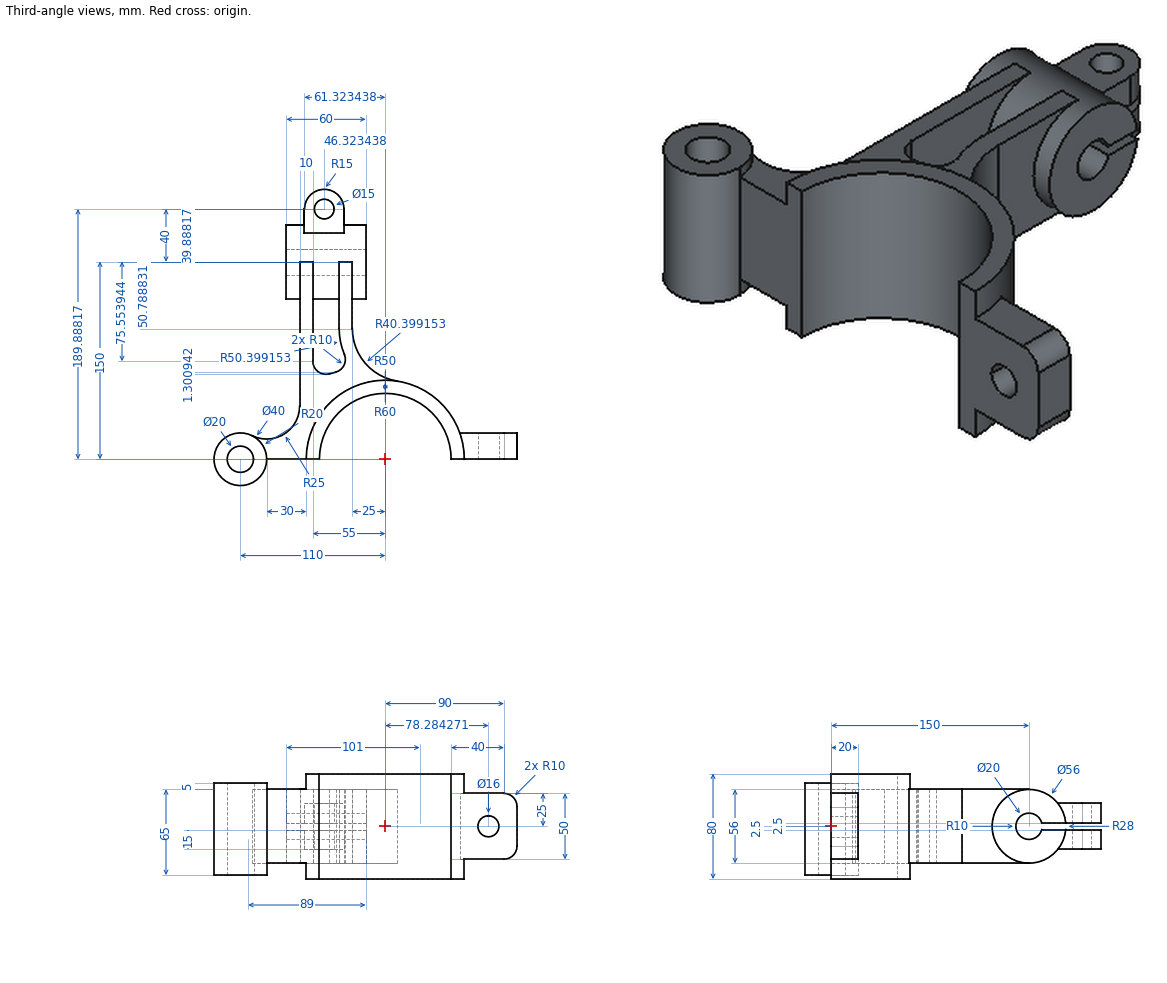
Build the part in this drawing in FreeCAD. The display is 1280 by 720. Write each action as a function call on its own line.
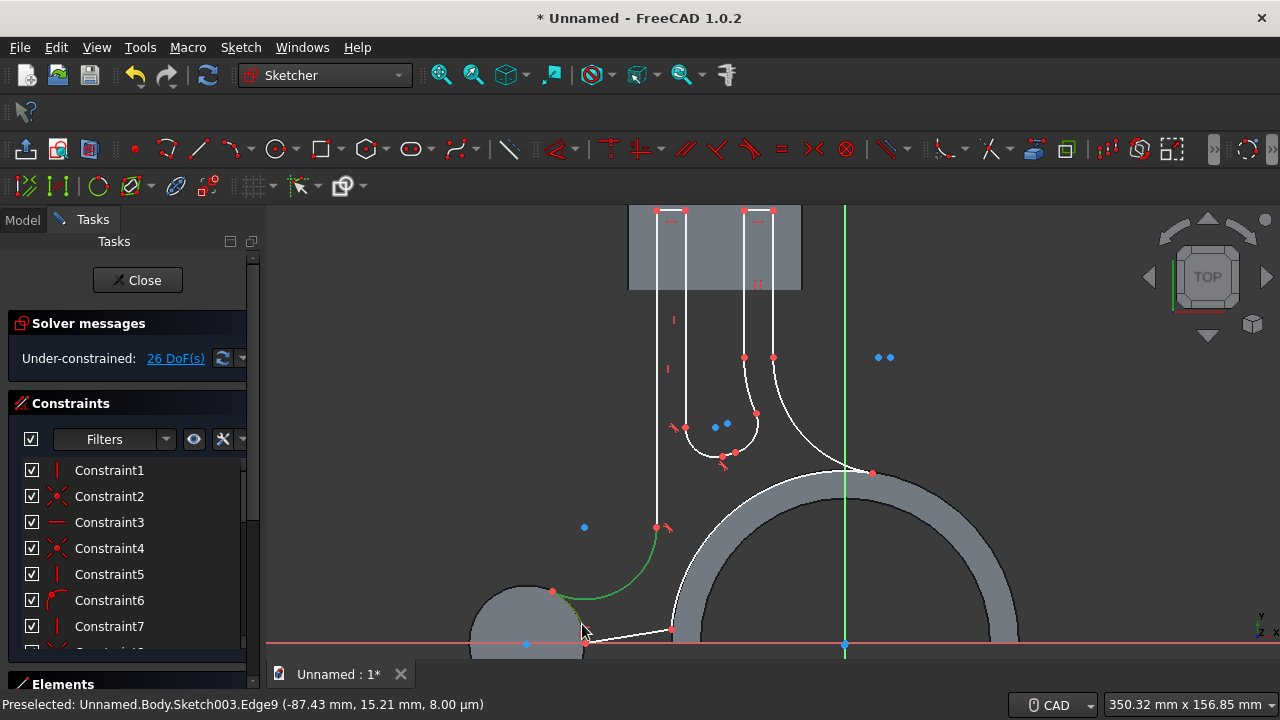
key(t)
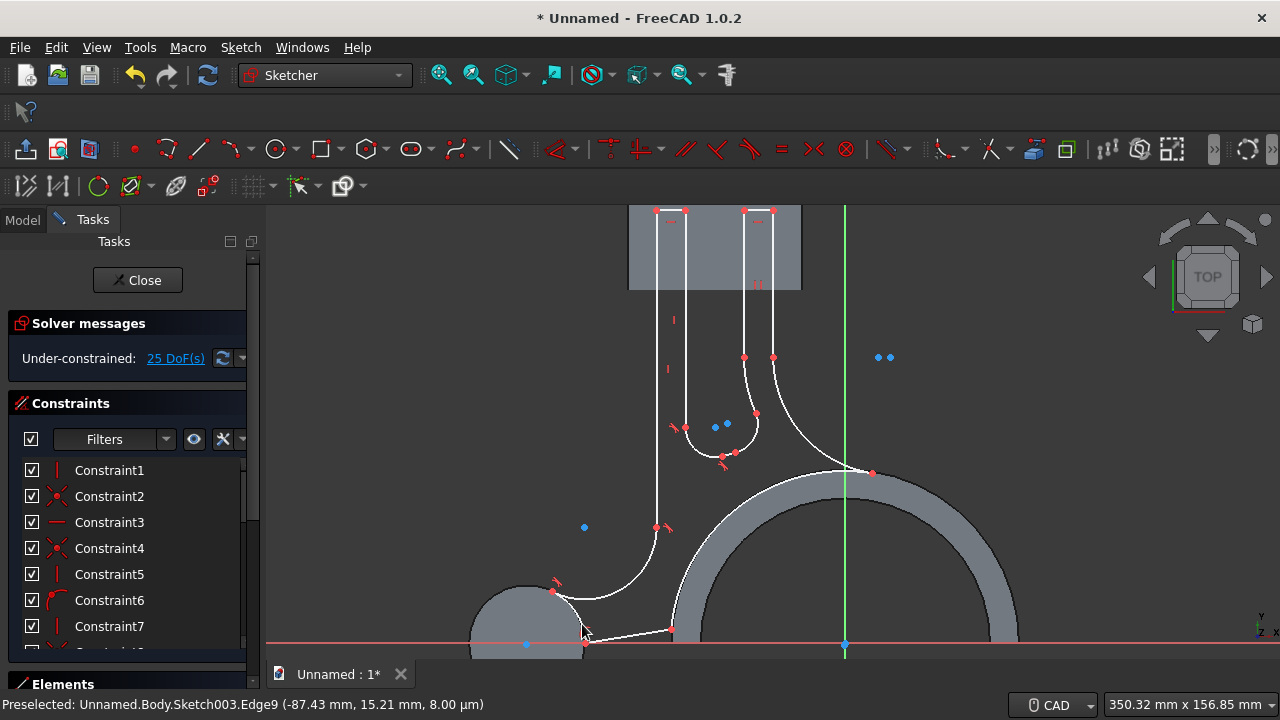
click(788, 481)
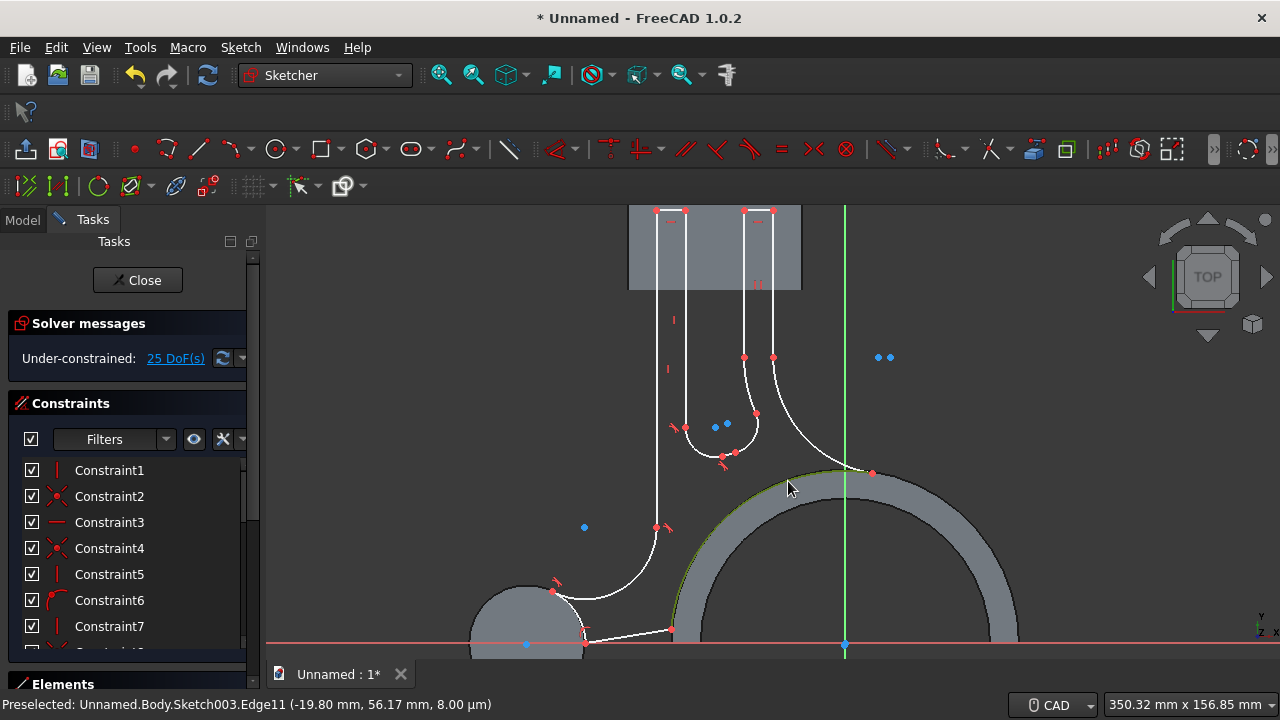
click(784, 406)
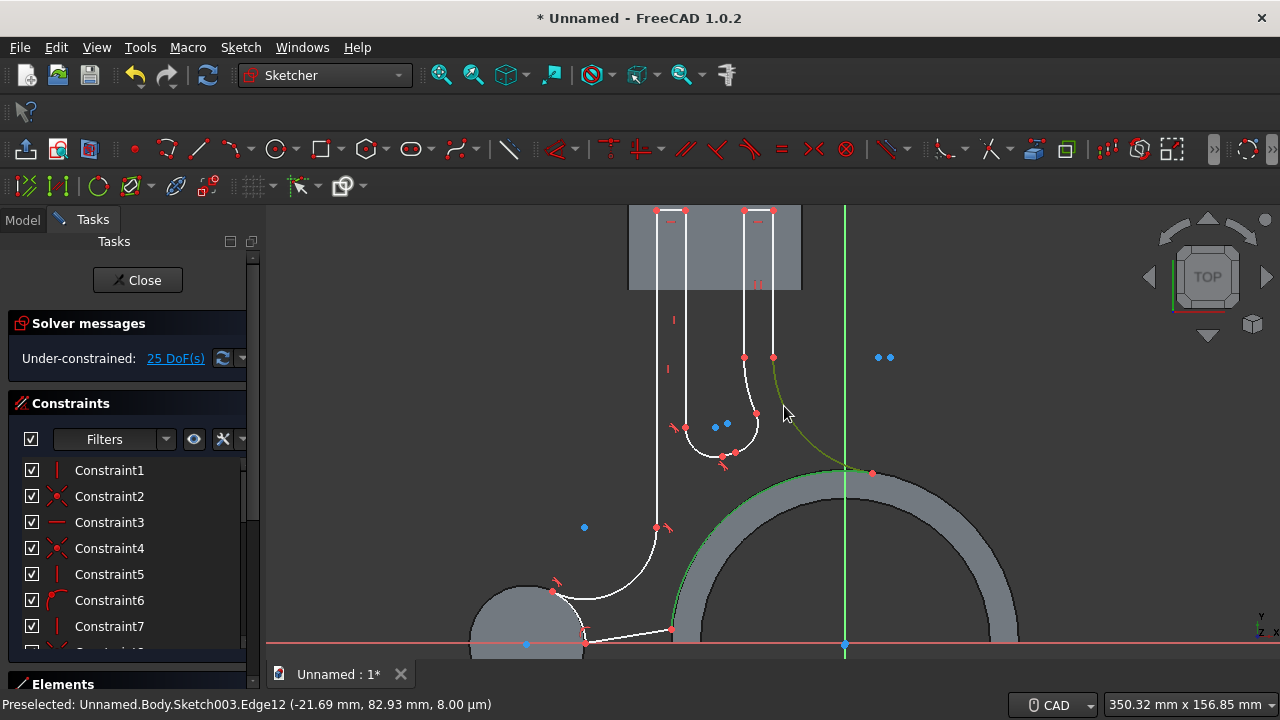
click(750, 150)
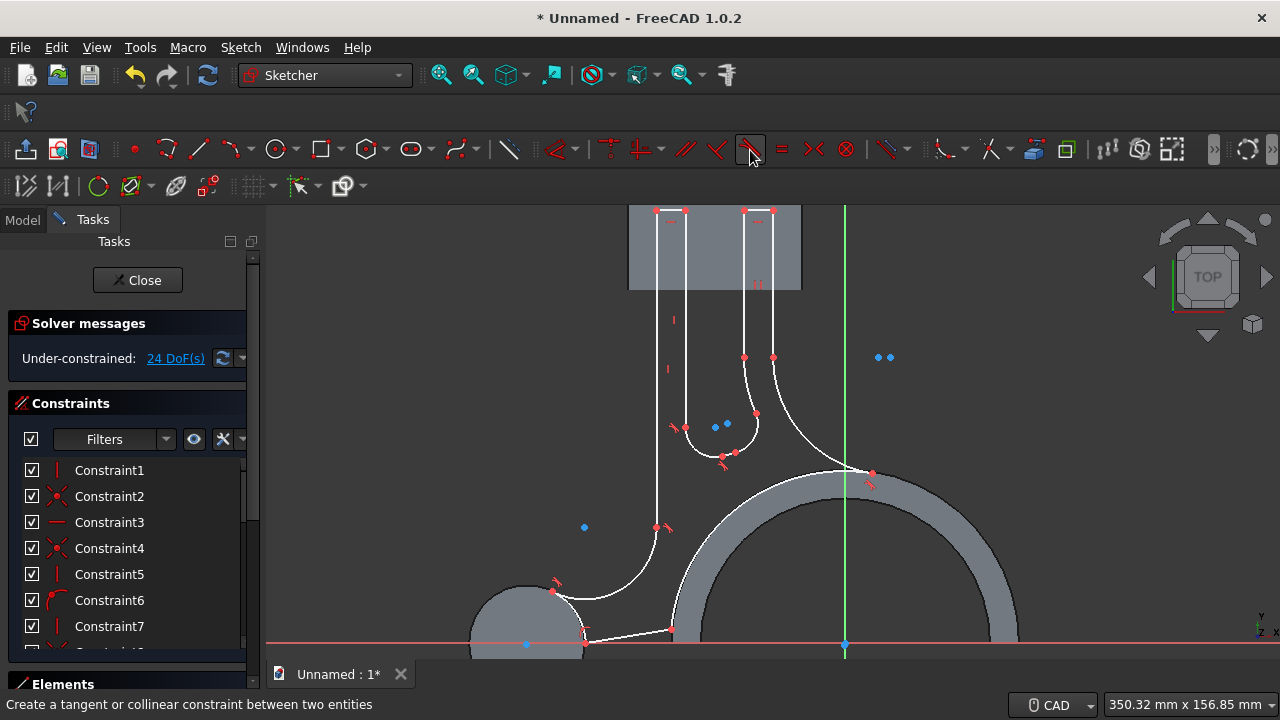
click(745, 375)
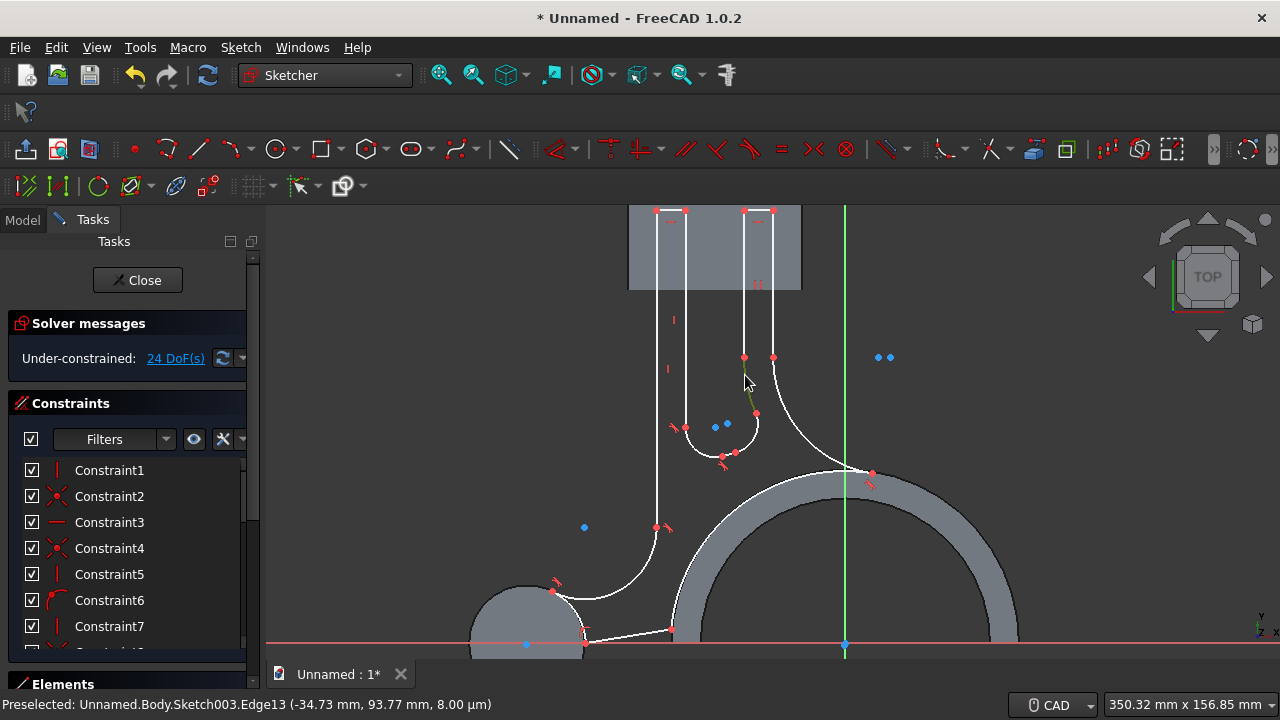
click(748, 446)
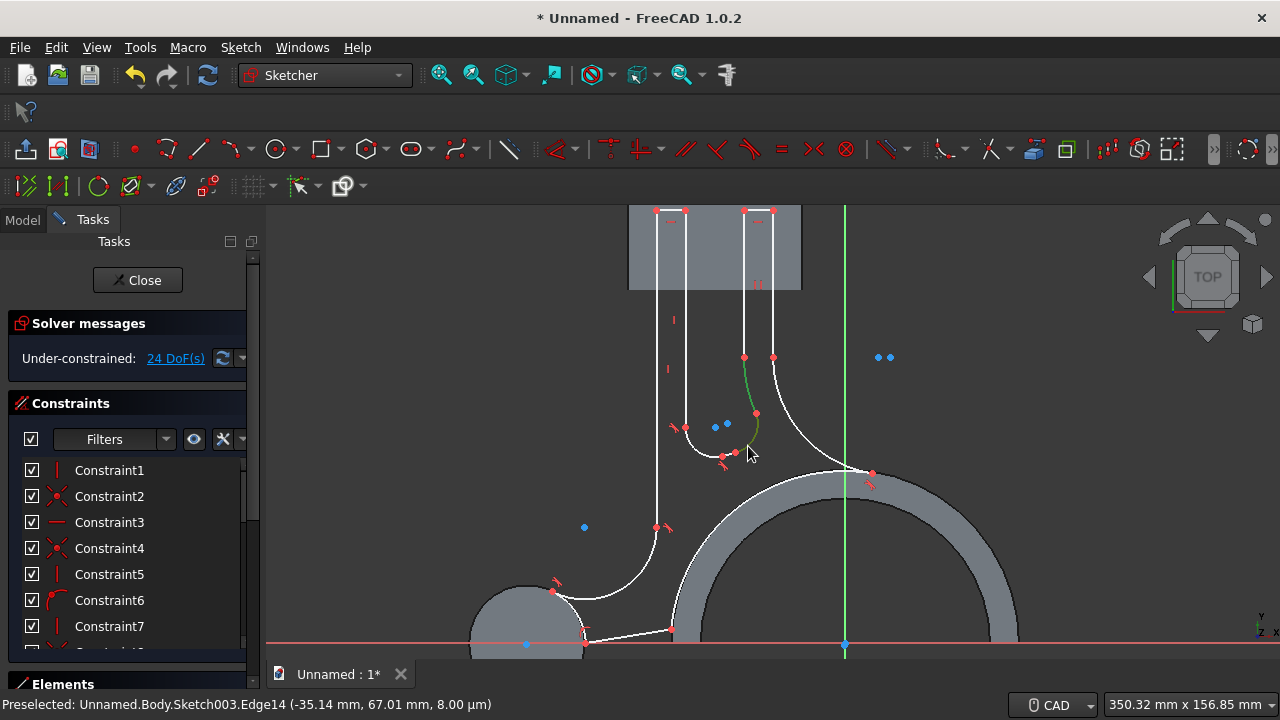
key(t)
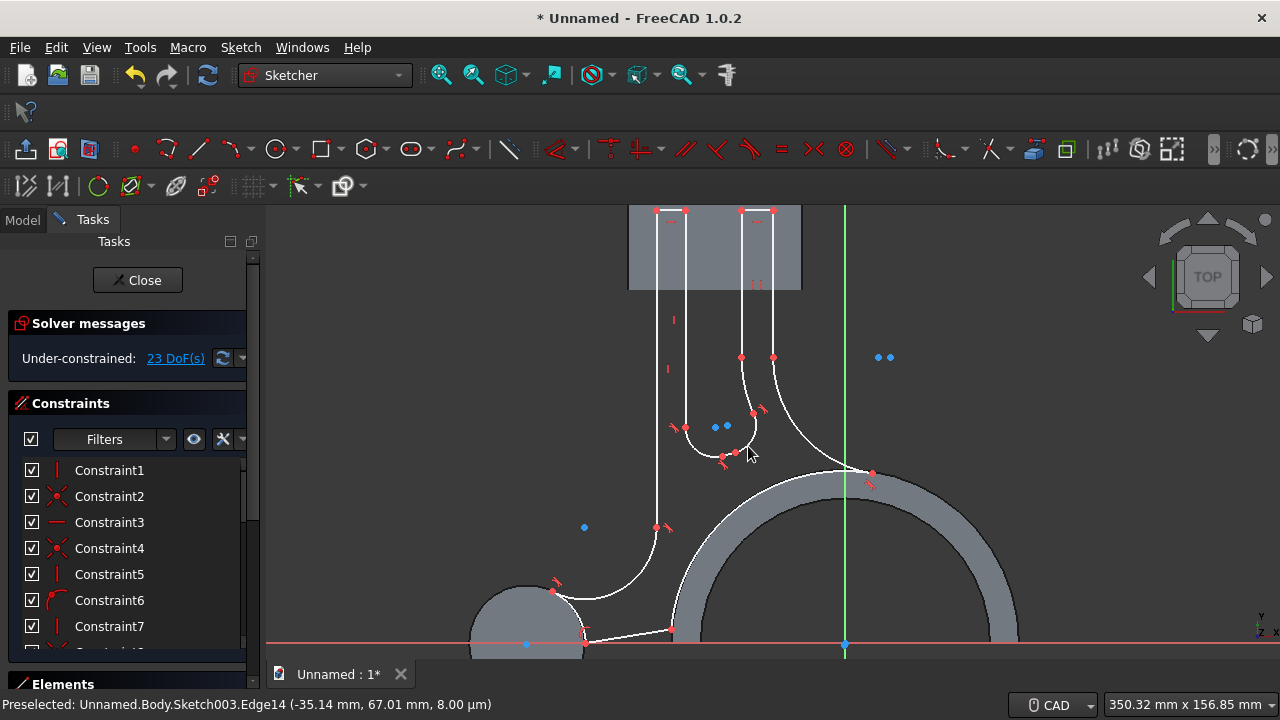
scroll(689, 444, down, 2)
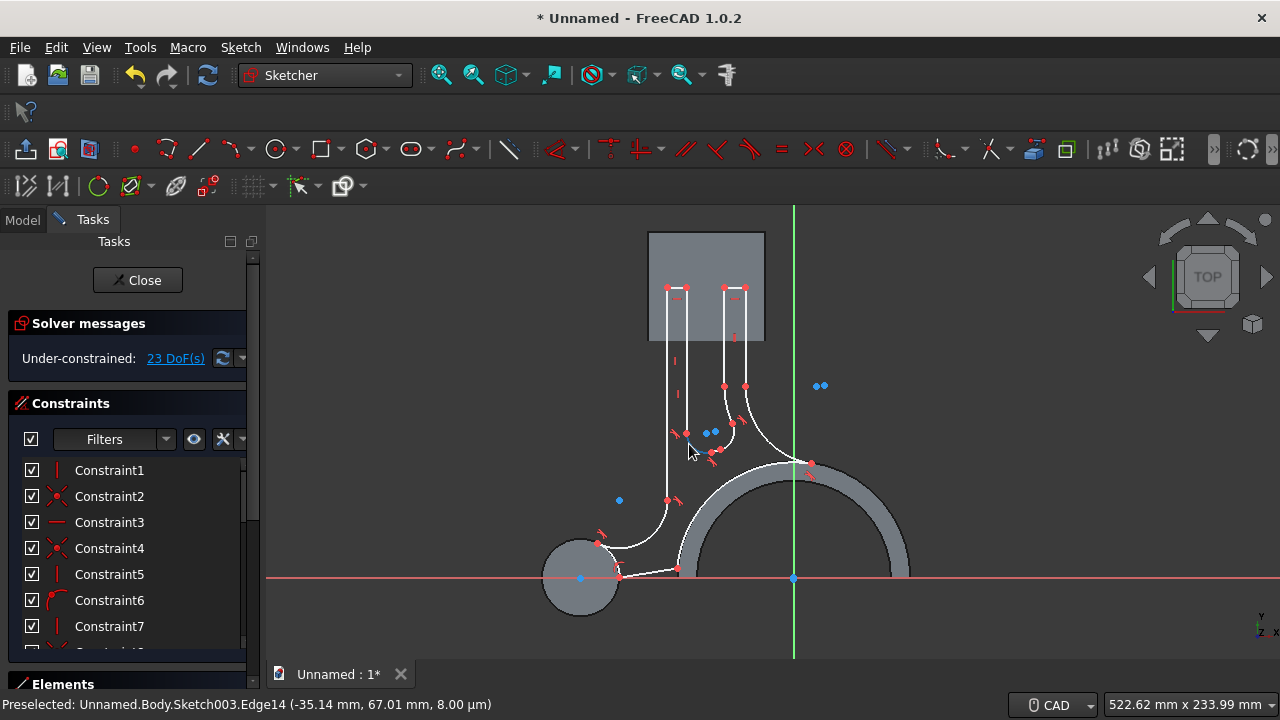
scroll(660, 571, up, 4)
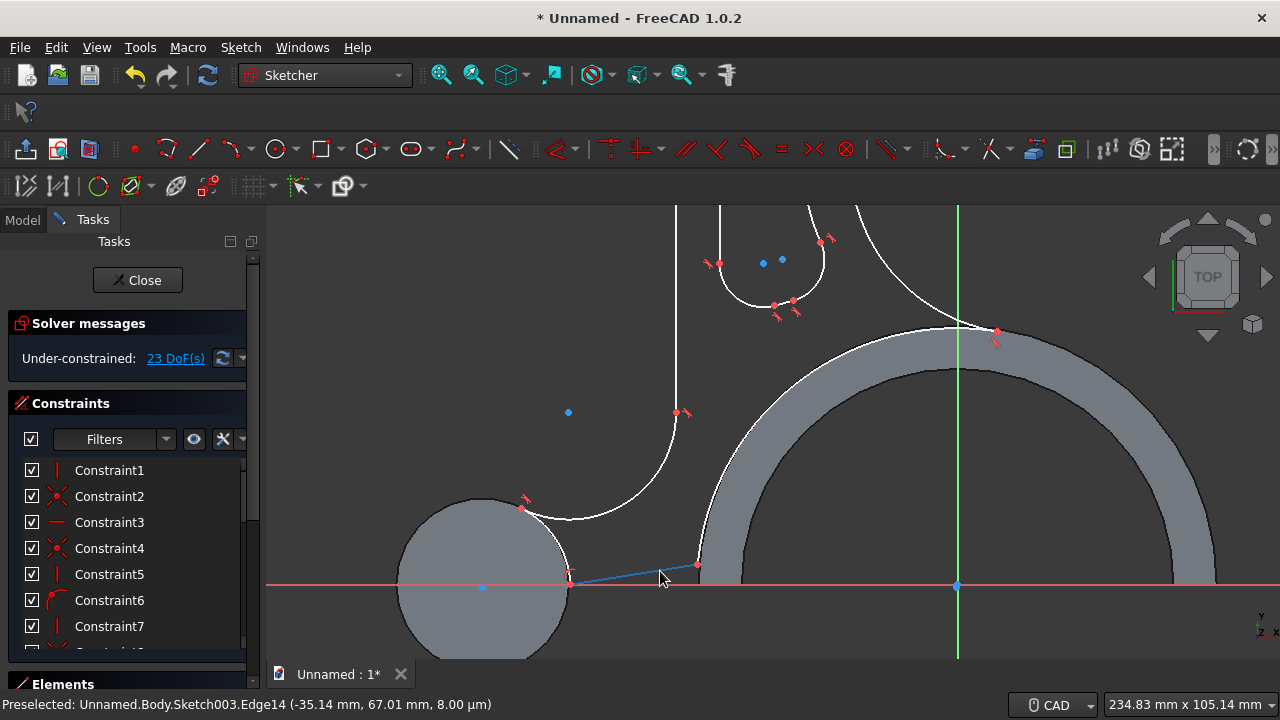
click(660, 570)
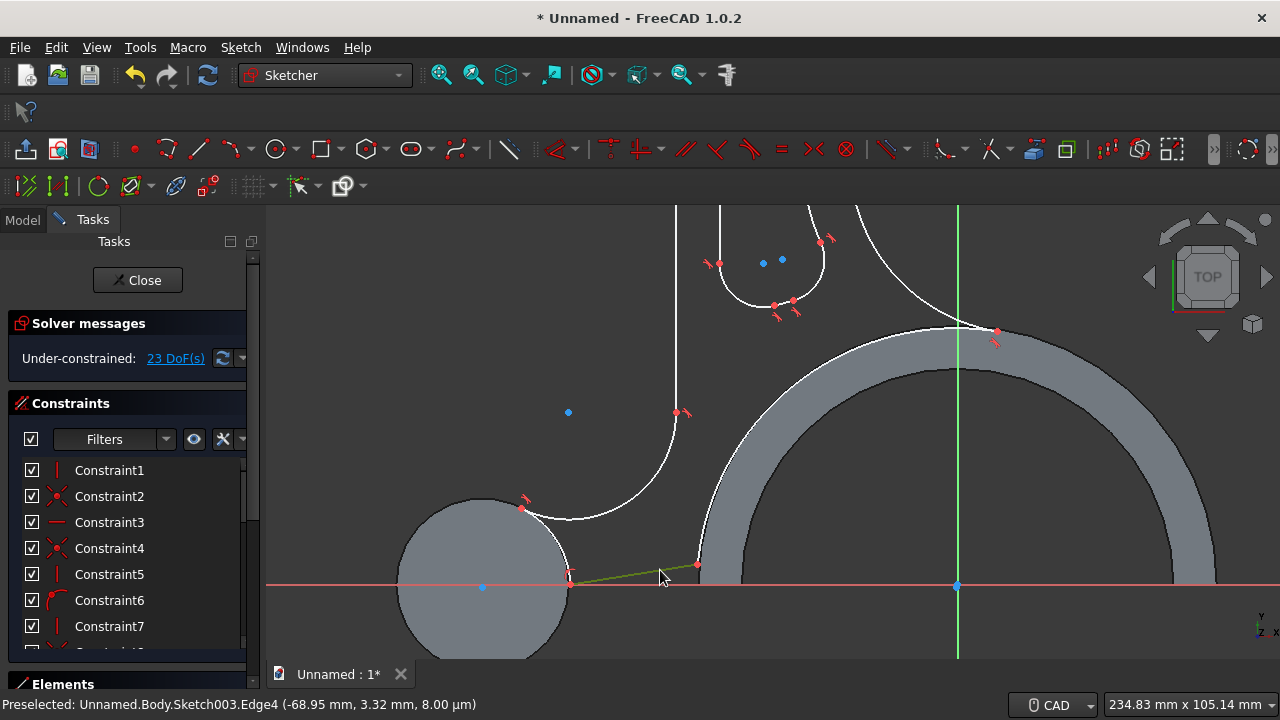
key(h)